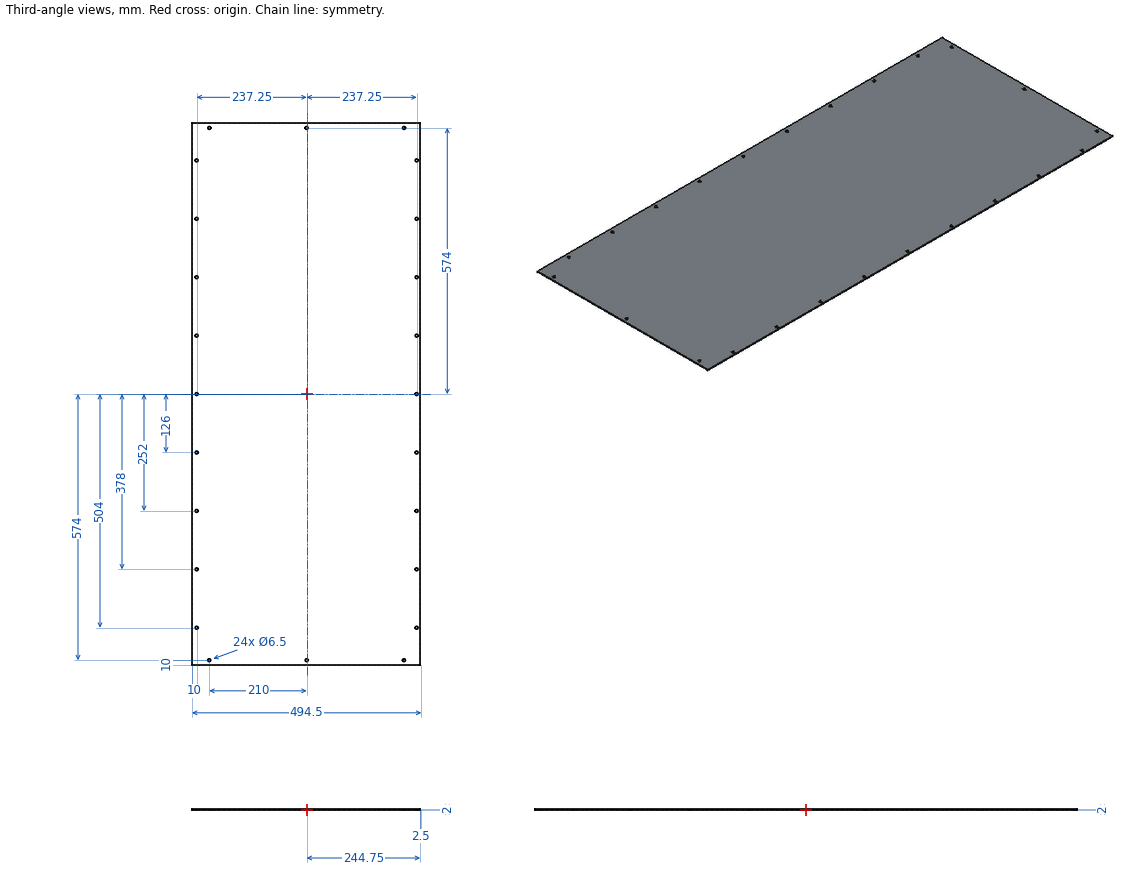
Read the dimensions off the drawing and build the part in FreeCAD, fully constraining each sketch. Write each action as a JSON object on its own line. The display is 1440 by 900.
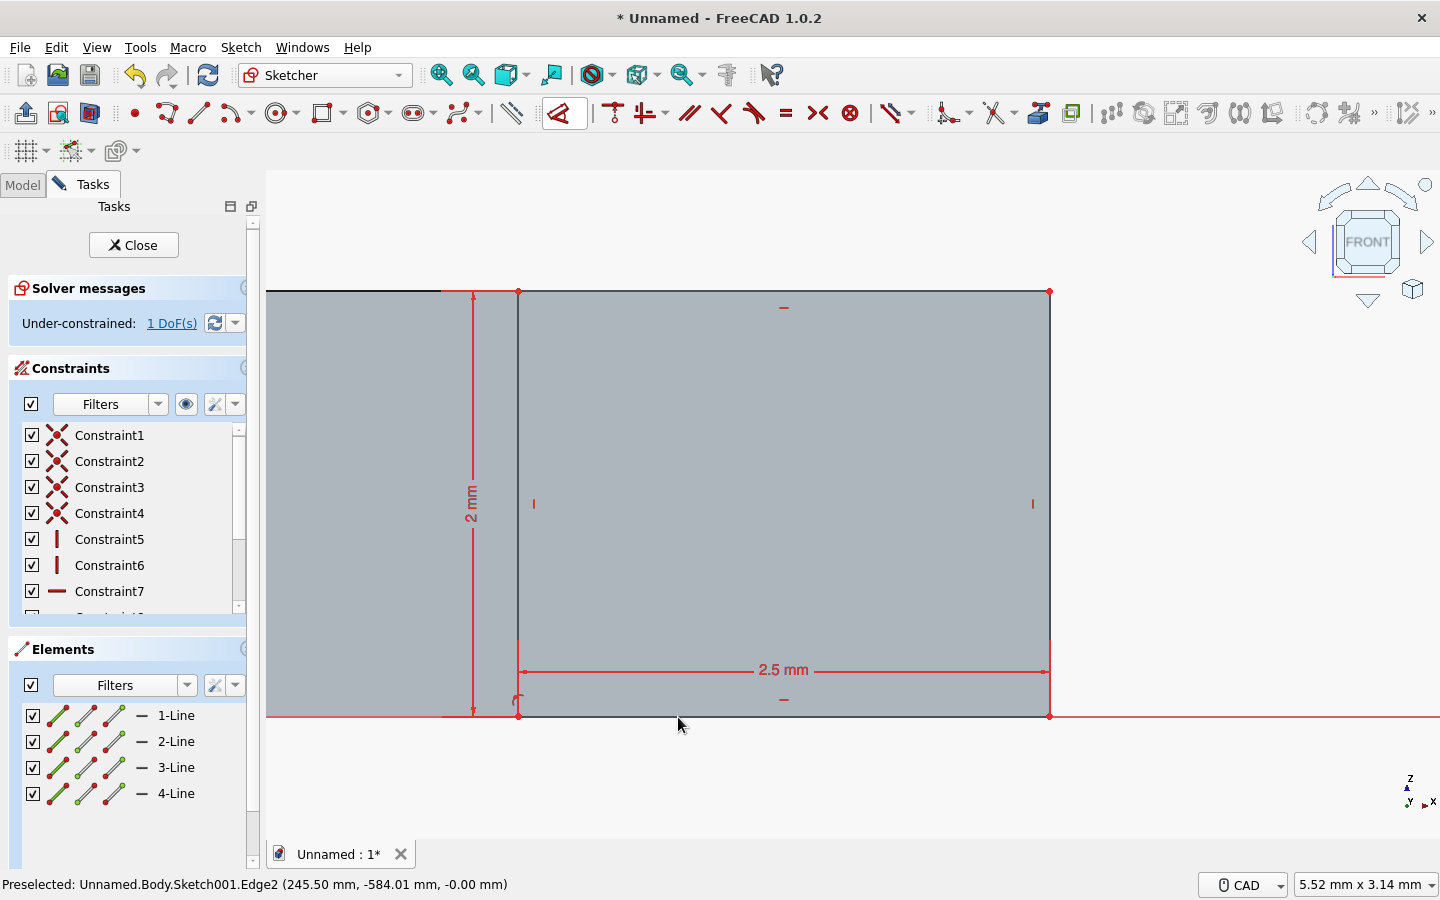
{"action": "left_click", "coordinate": [518, 291]}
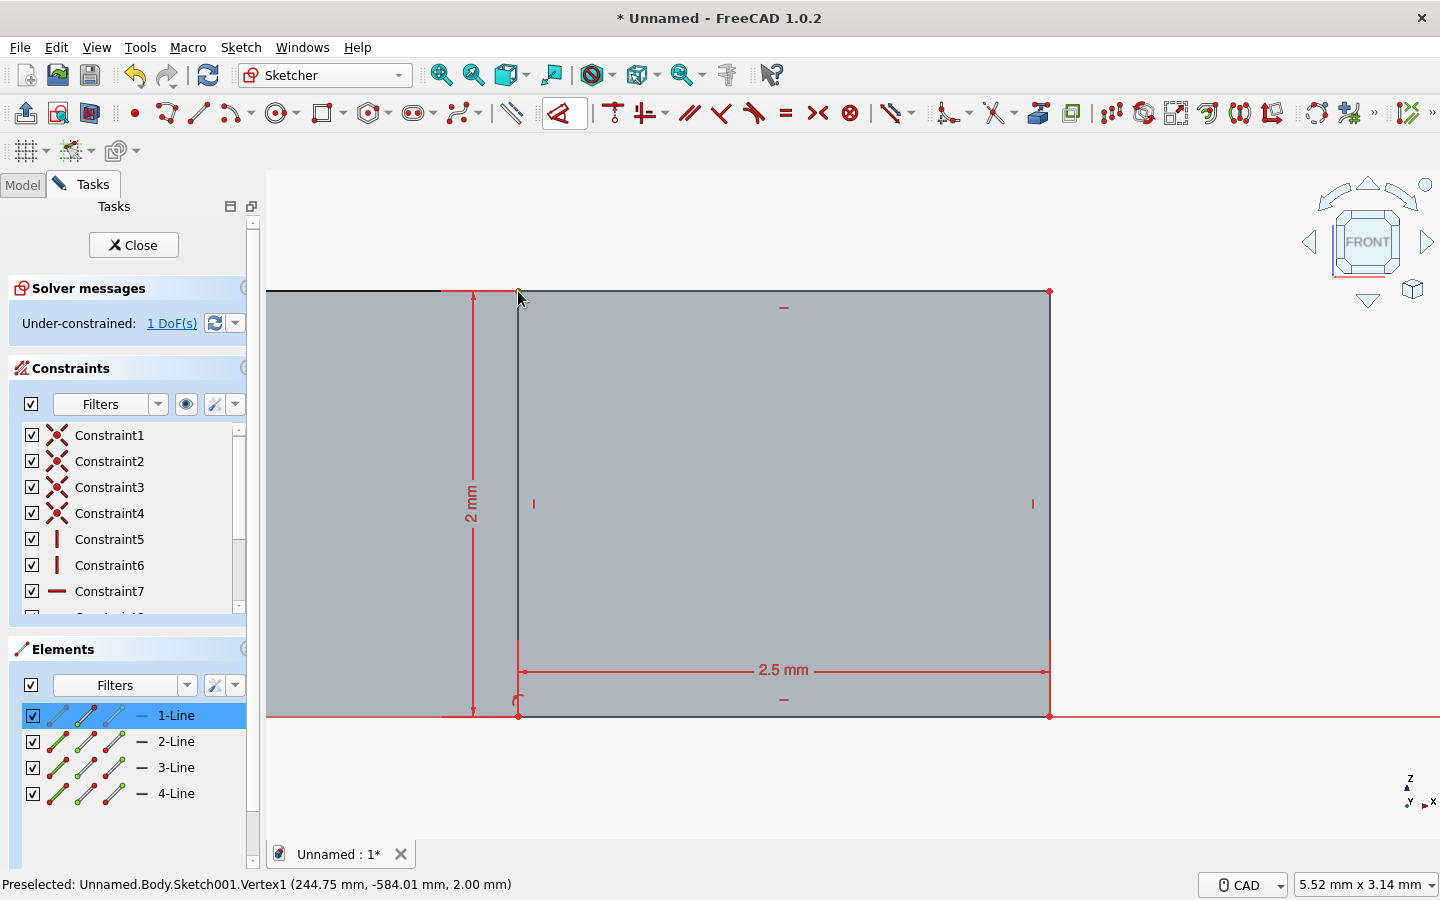
{"action": "key", "text": "l"}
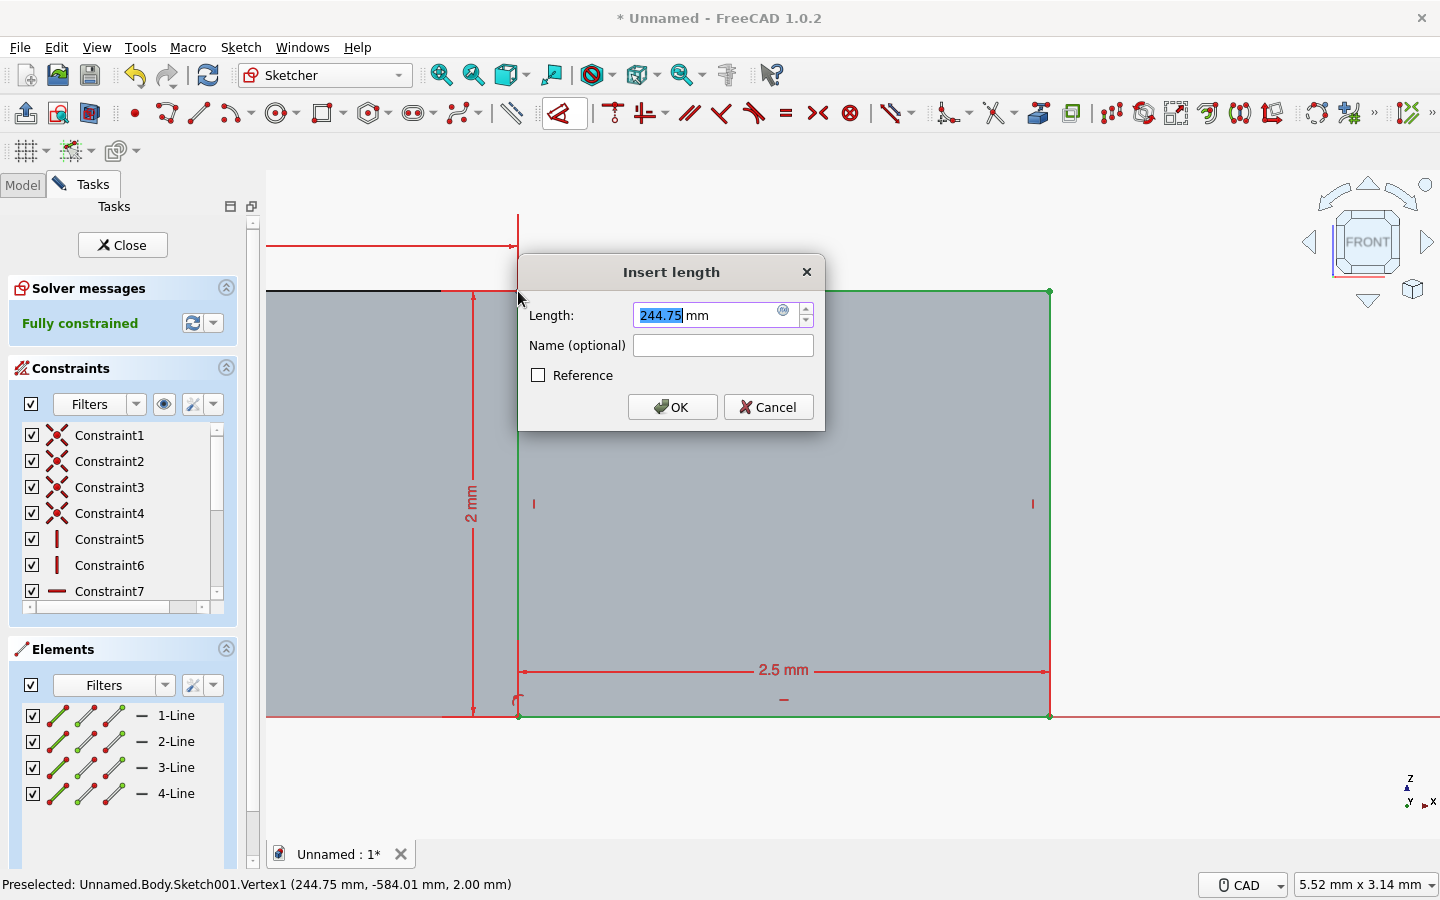
{"action": "type", "text": "244.75"}
{"action": "key", "text": "Return"}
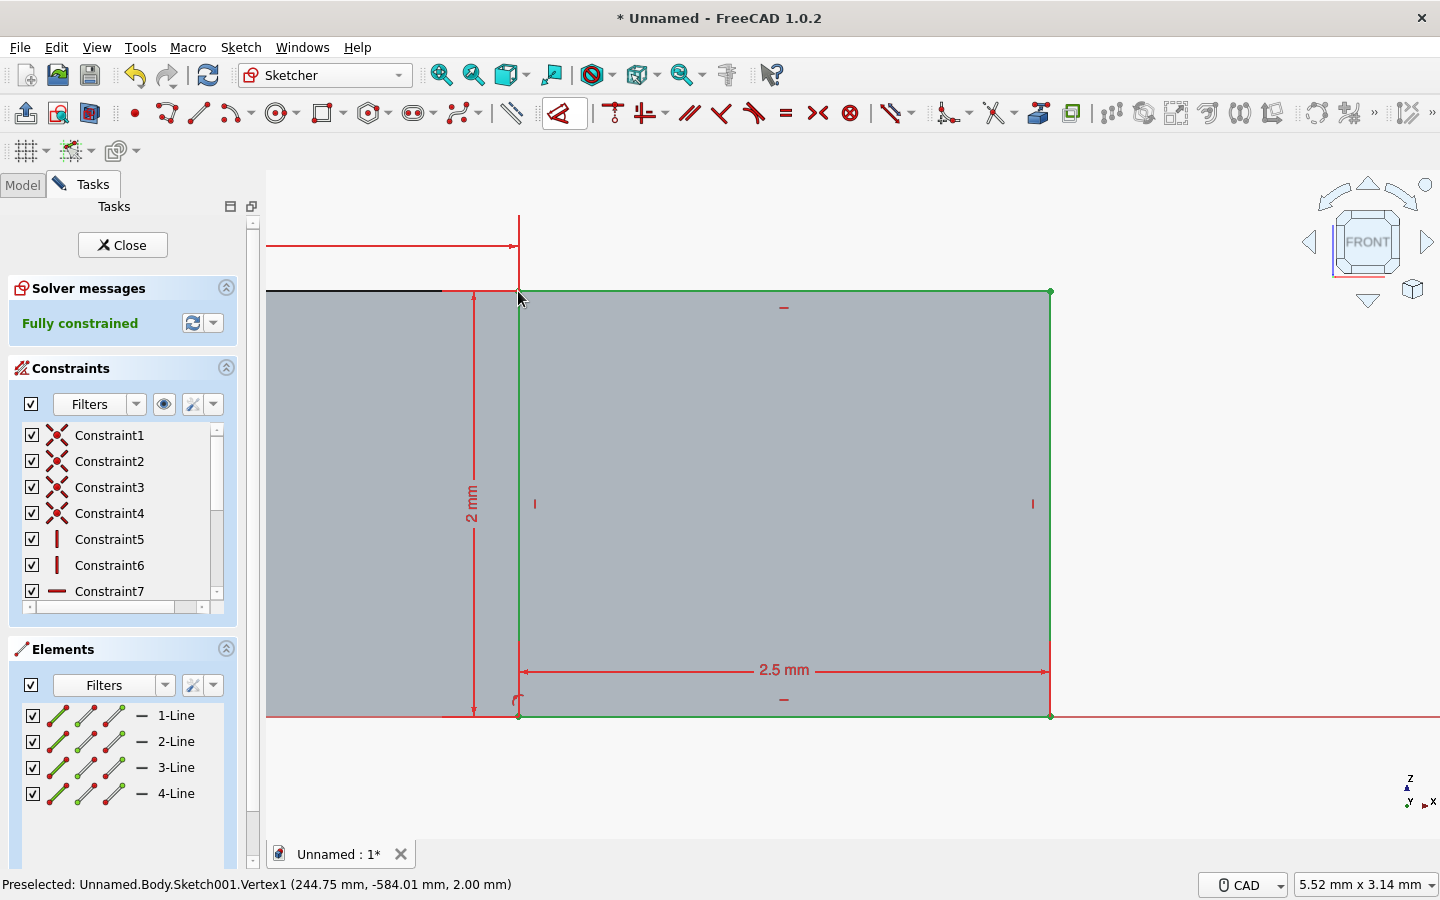
{"action": "left_click", "coordinate": [123, 245]}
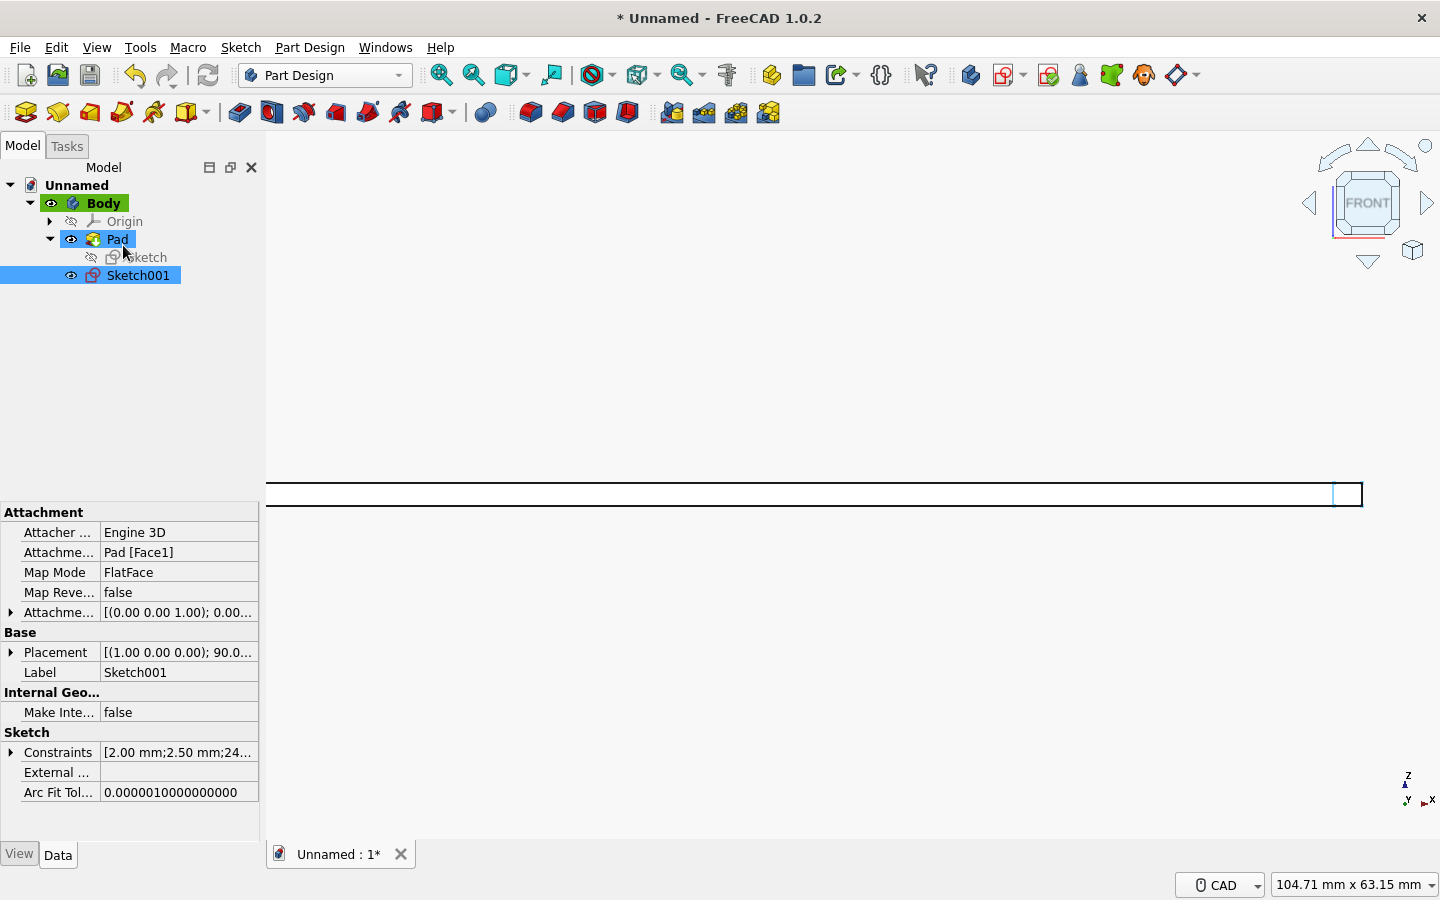
{"action": "left_click", "coordinate": [240, 112]}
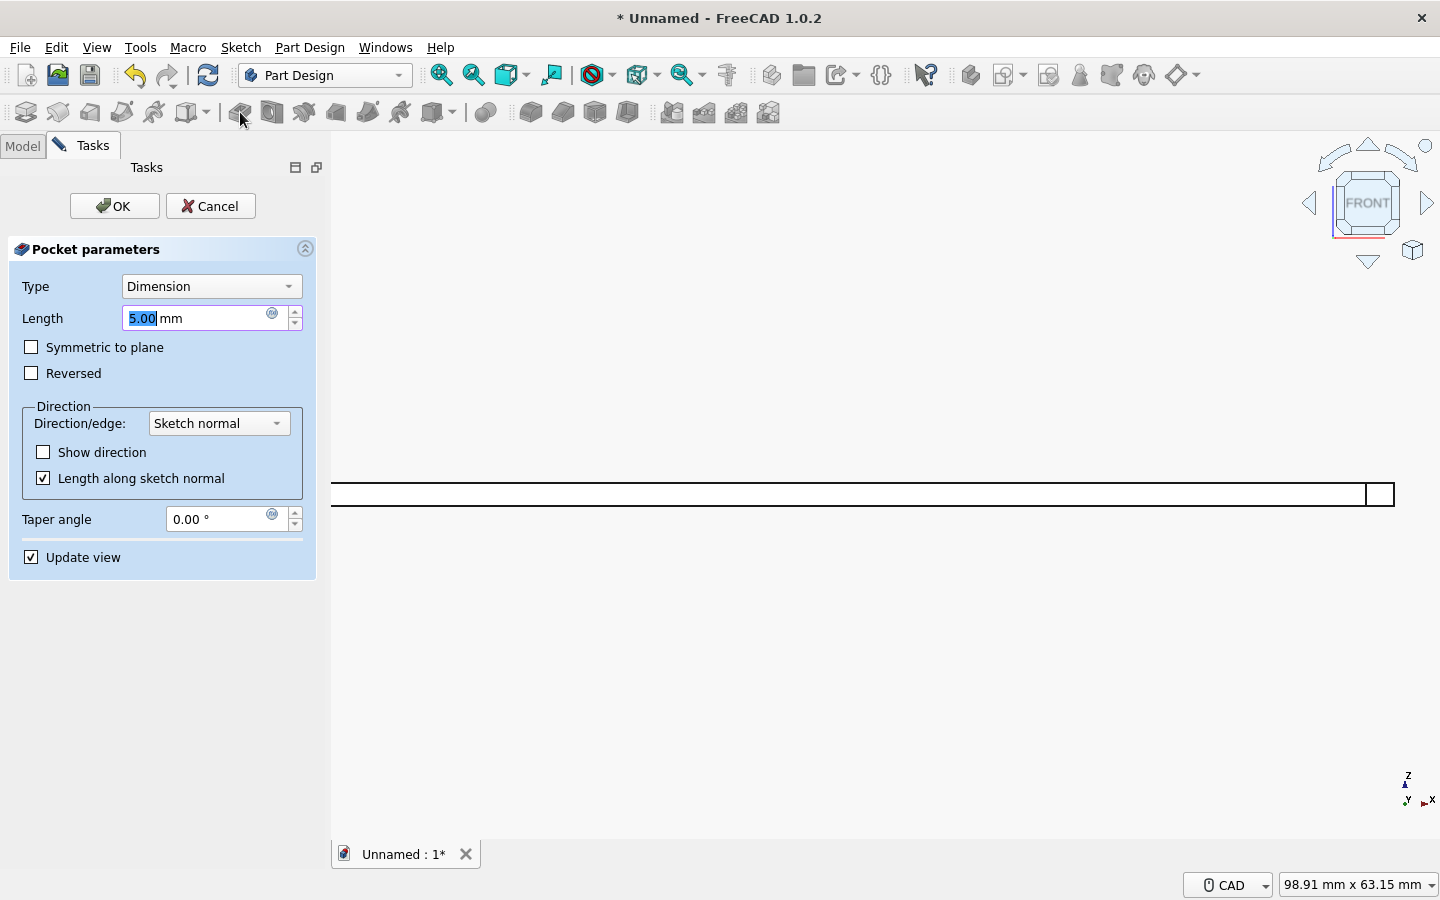
{"action": "left_click", "coordinate": [212, 286]}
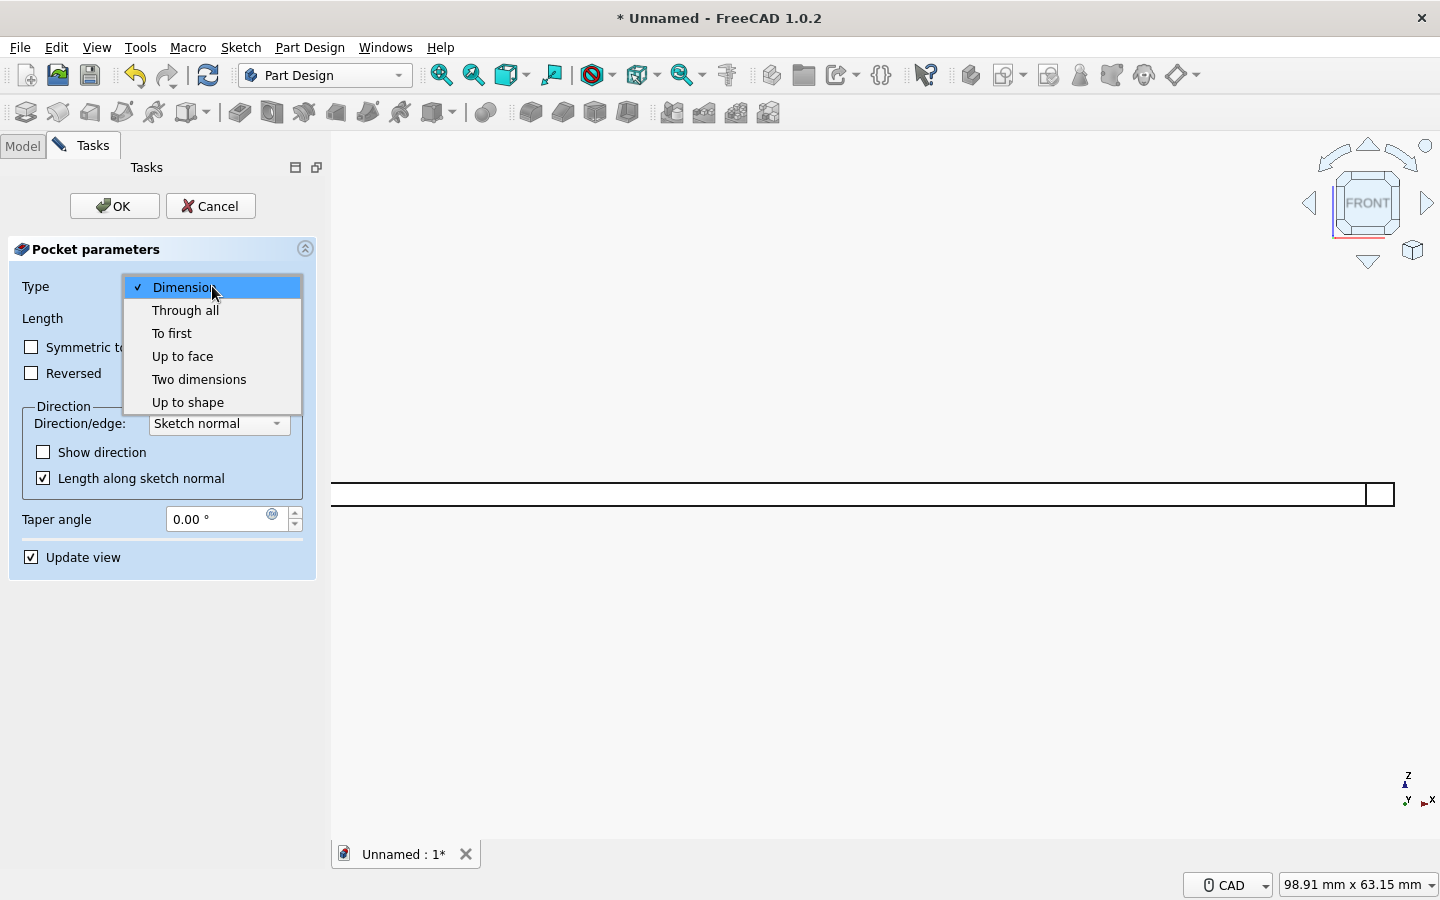
{"action": "left_click", "coordinate": [212, 310]}